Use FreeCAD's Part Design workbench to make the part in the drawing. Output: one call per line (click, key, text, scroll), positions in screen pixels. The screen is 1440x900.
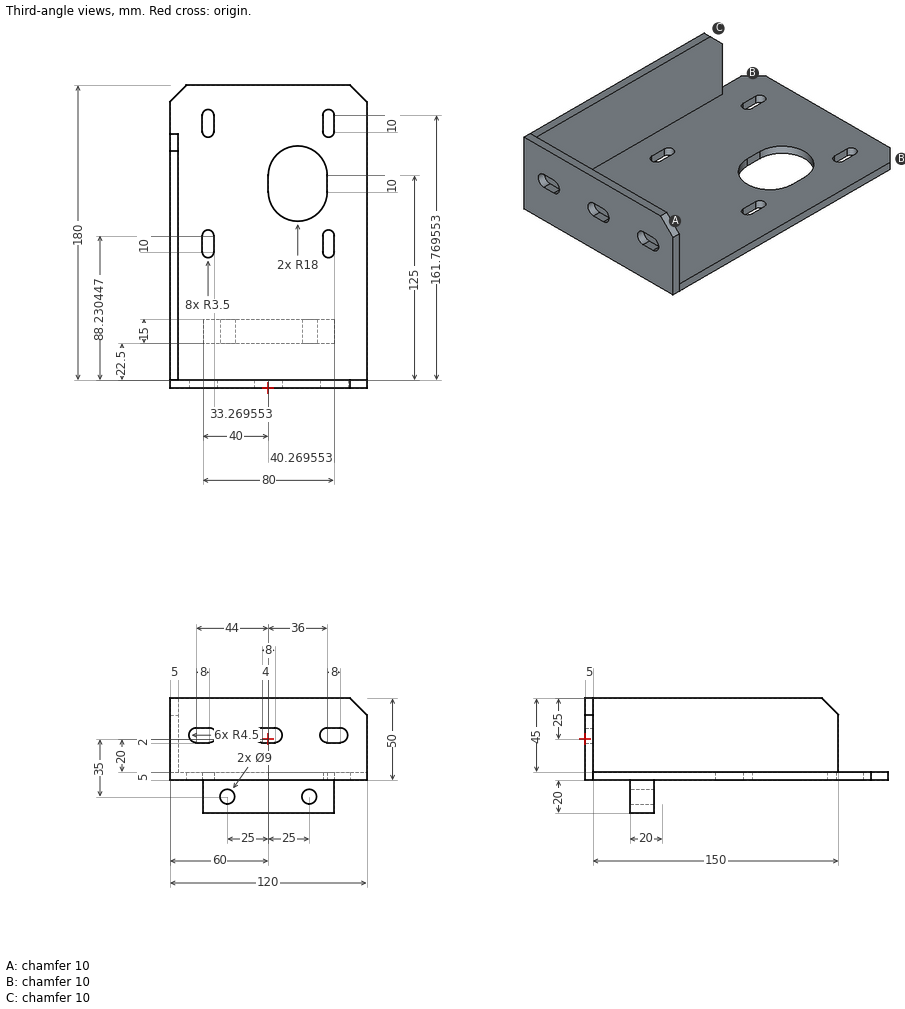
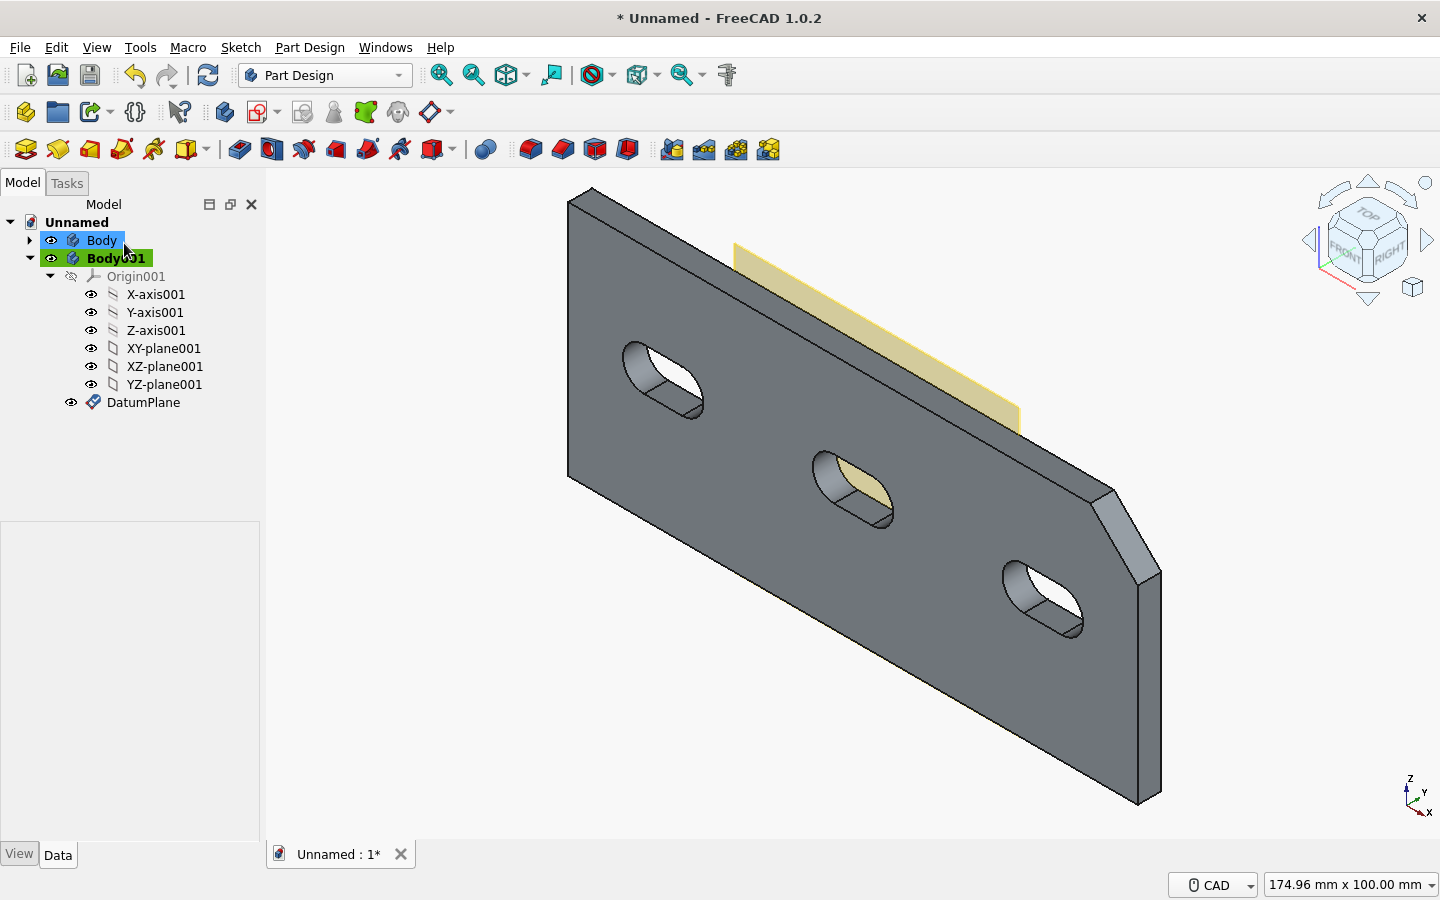
click(116, 402)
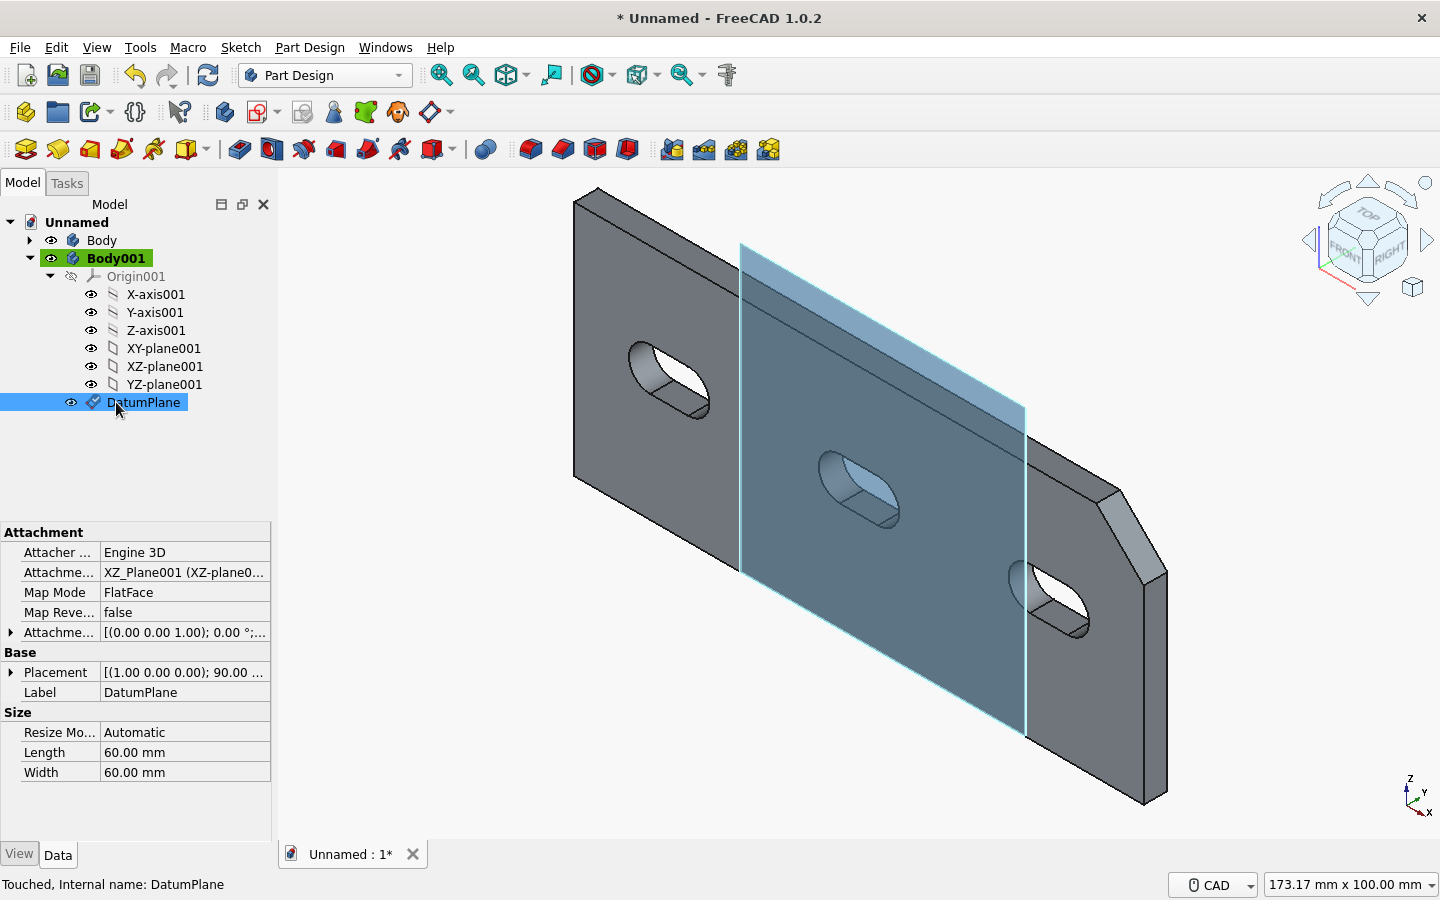
click(258, 112)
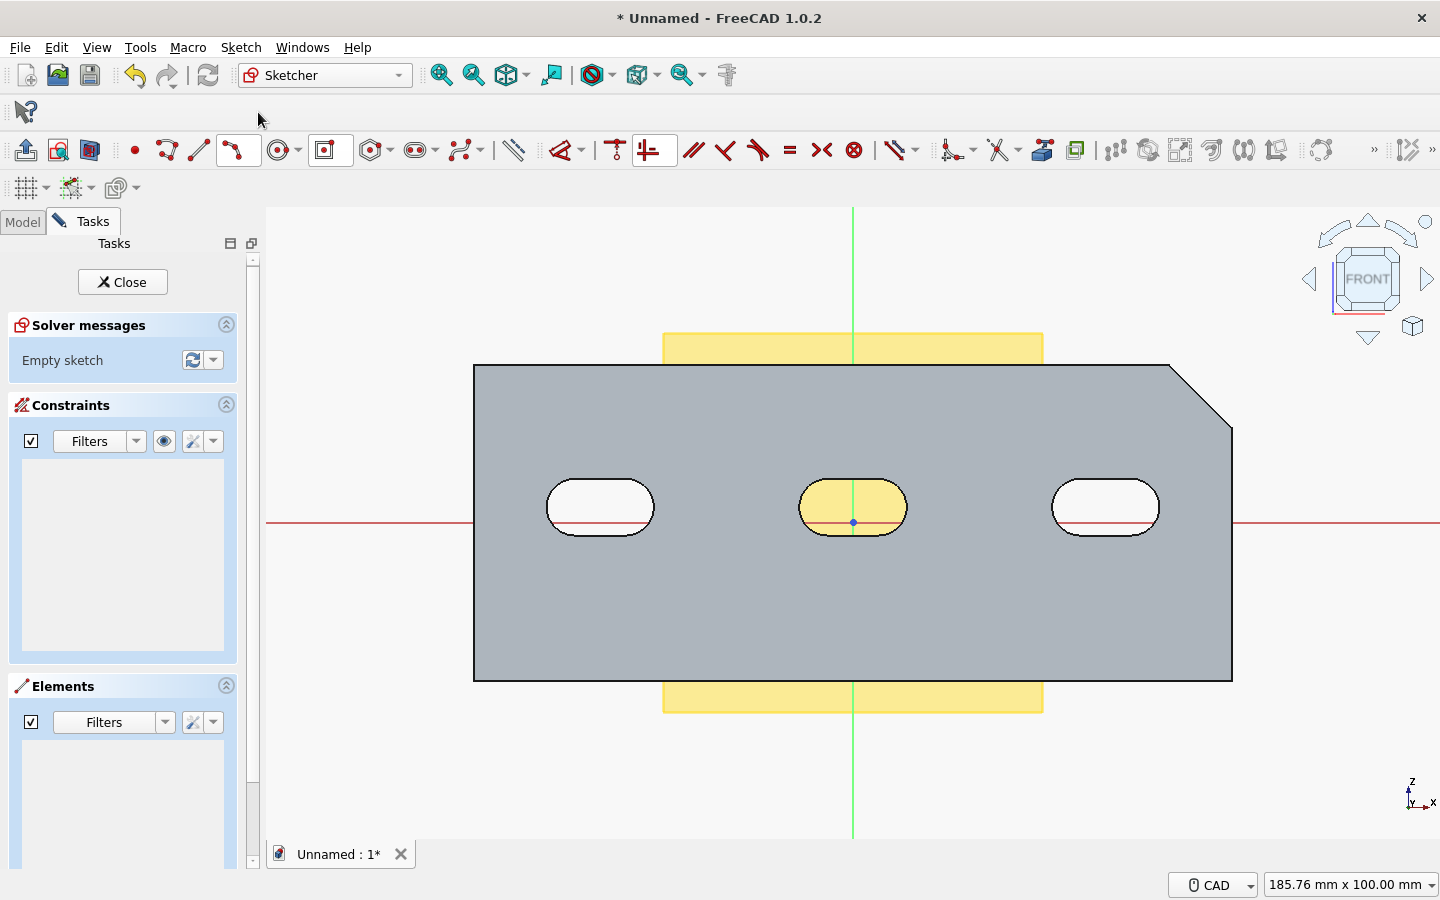
click(348, 150)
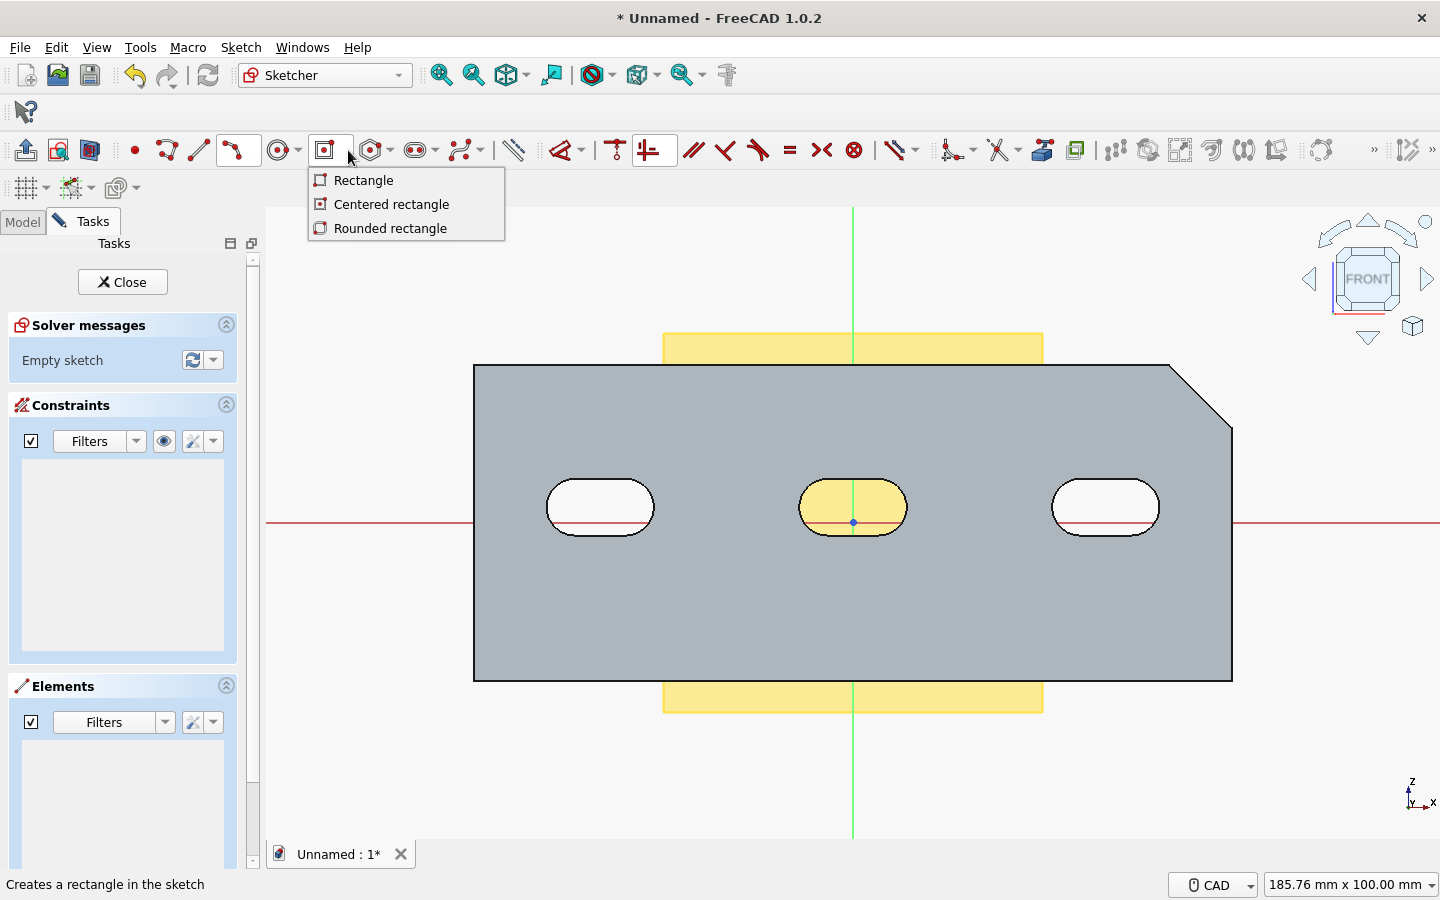
click(406, 180)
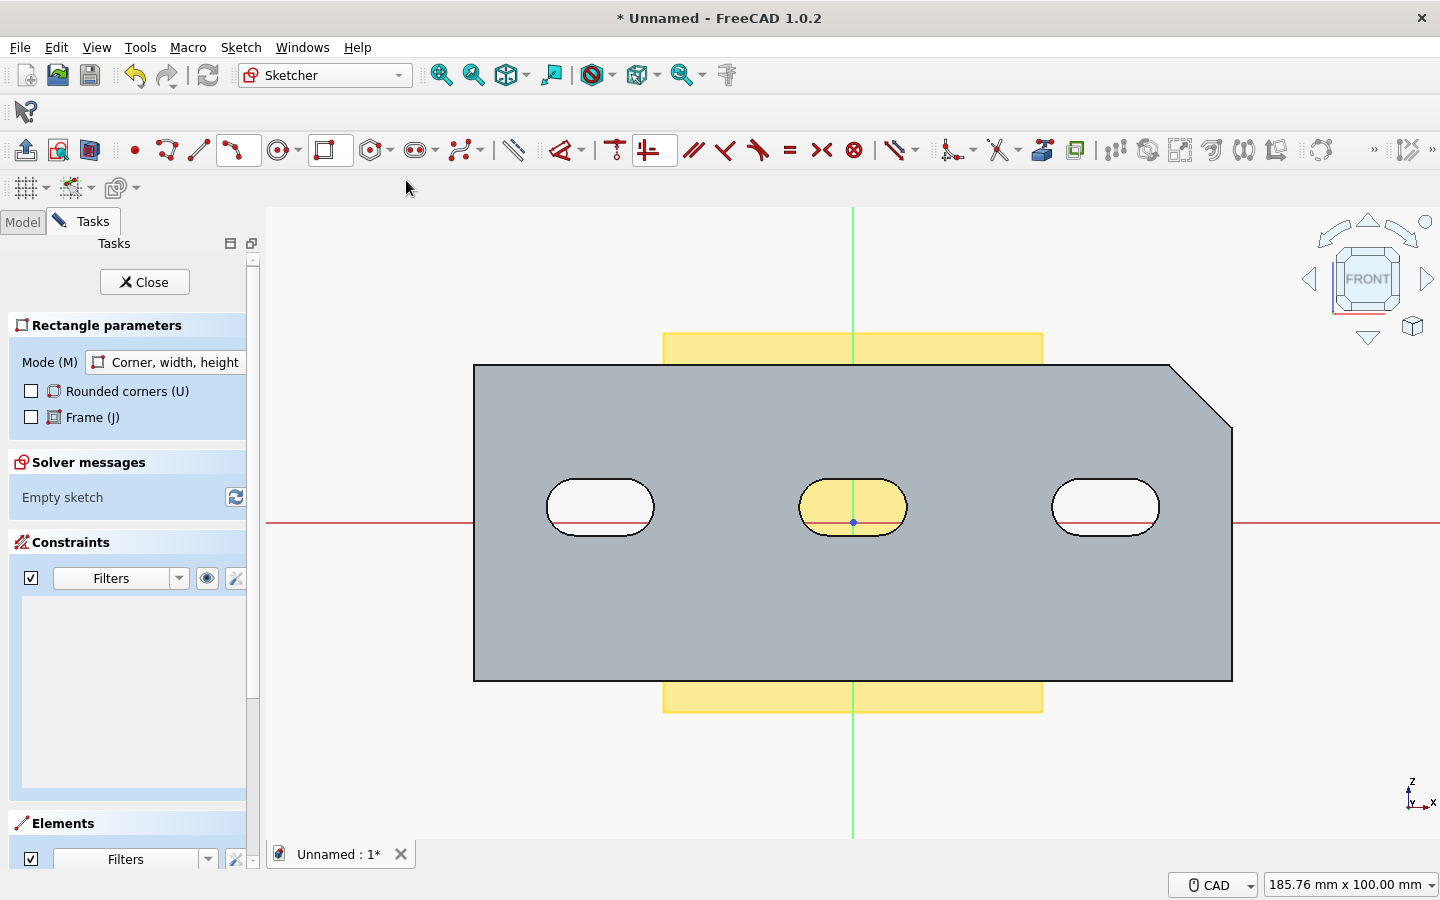
click(474, 649)
click(1232, 681)
key(Escape)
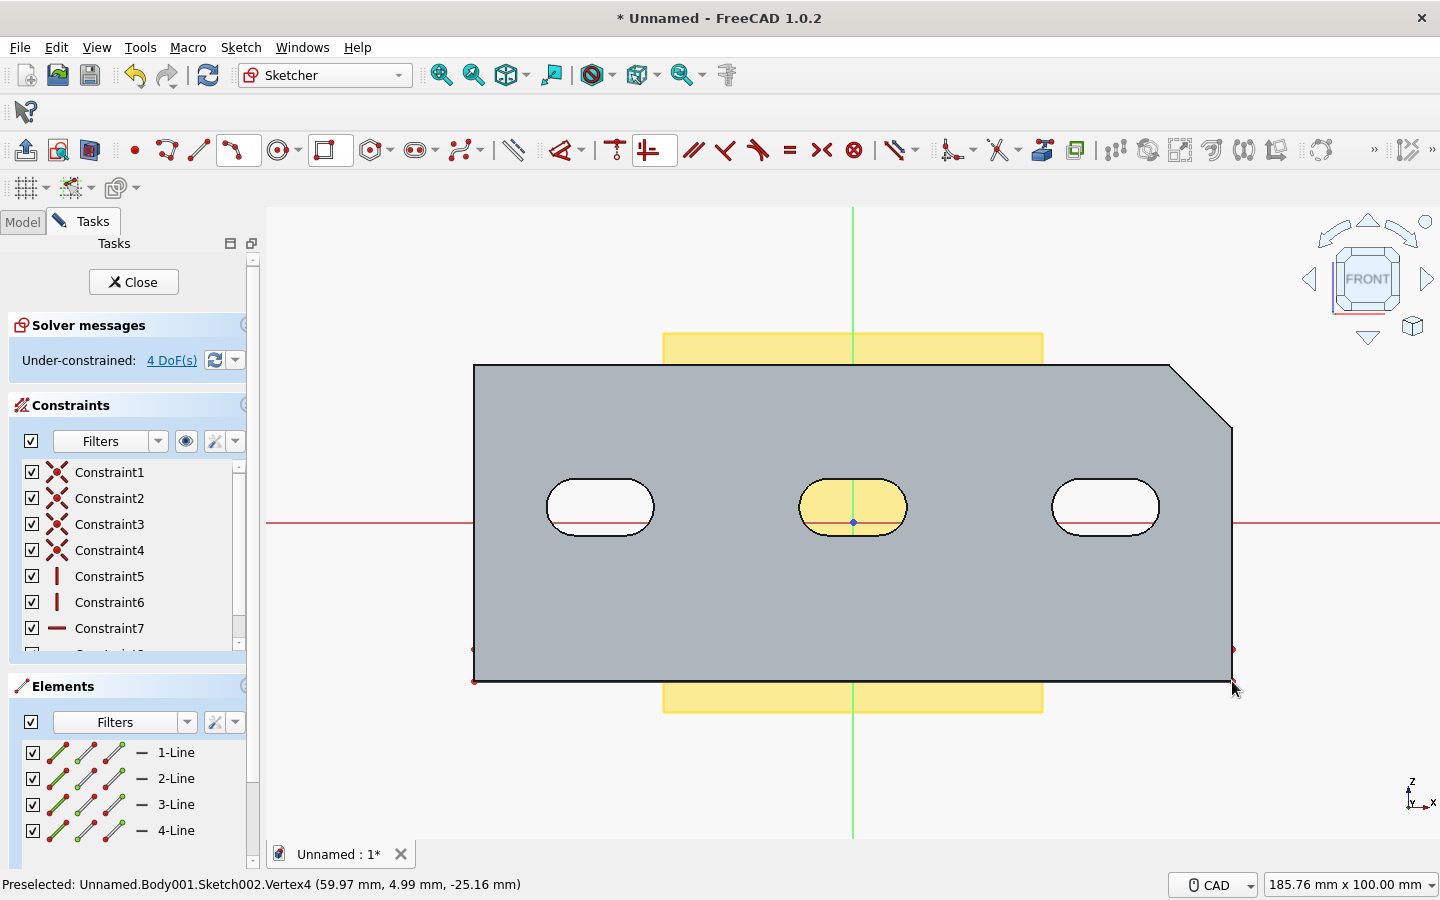
click(560, 150)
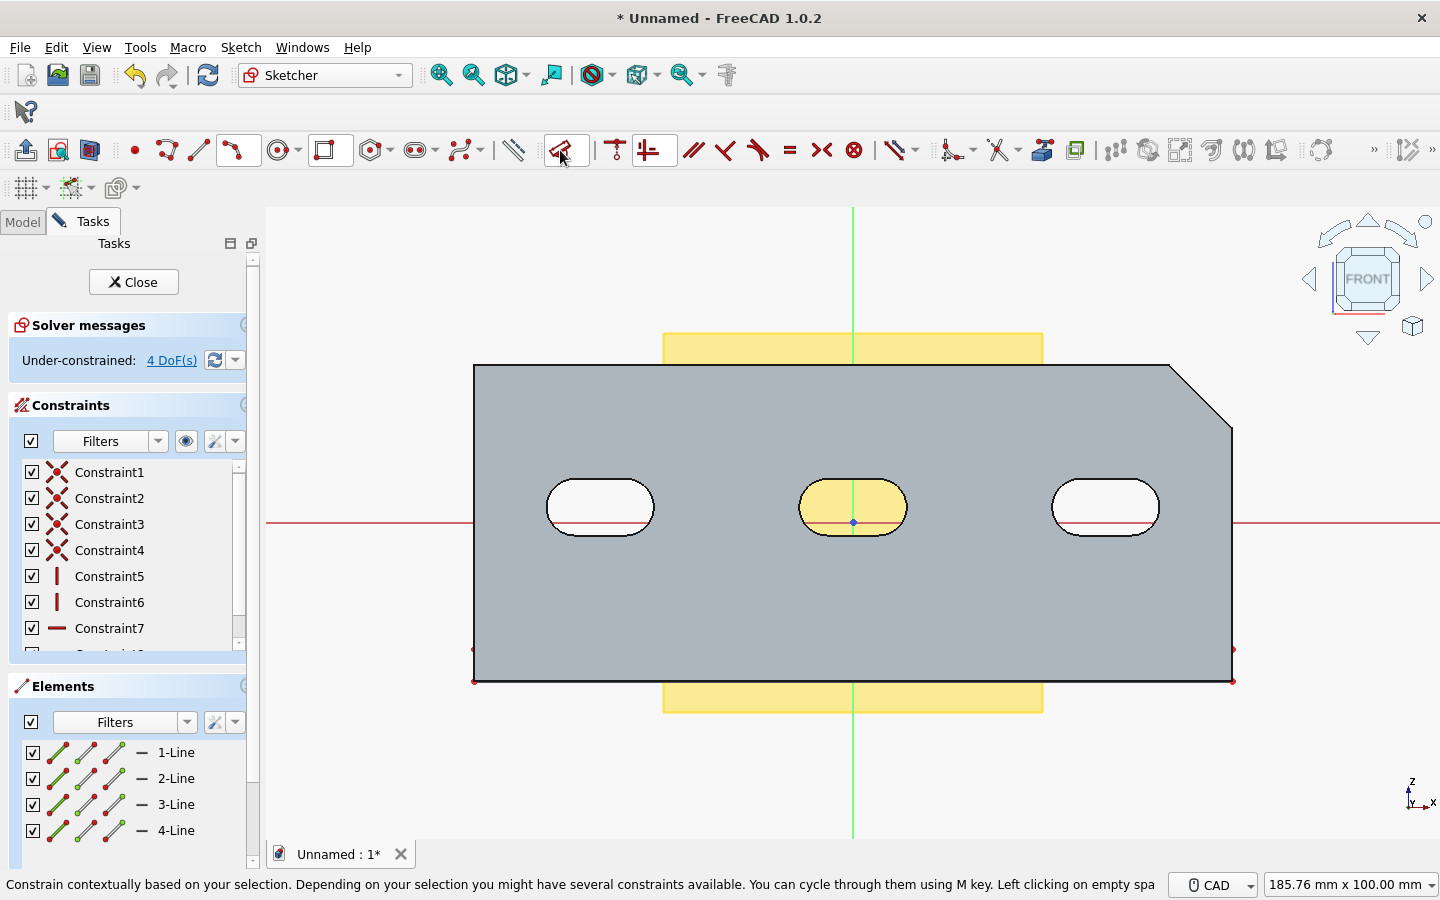
scroll(474, 660, up, 2)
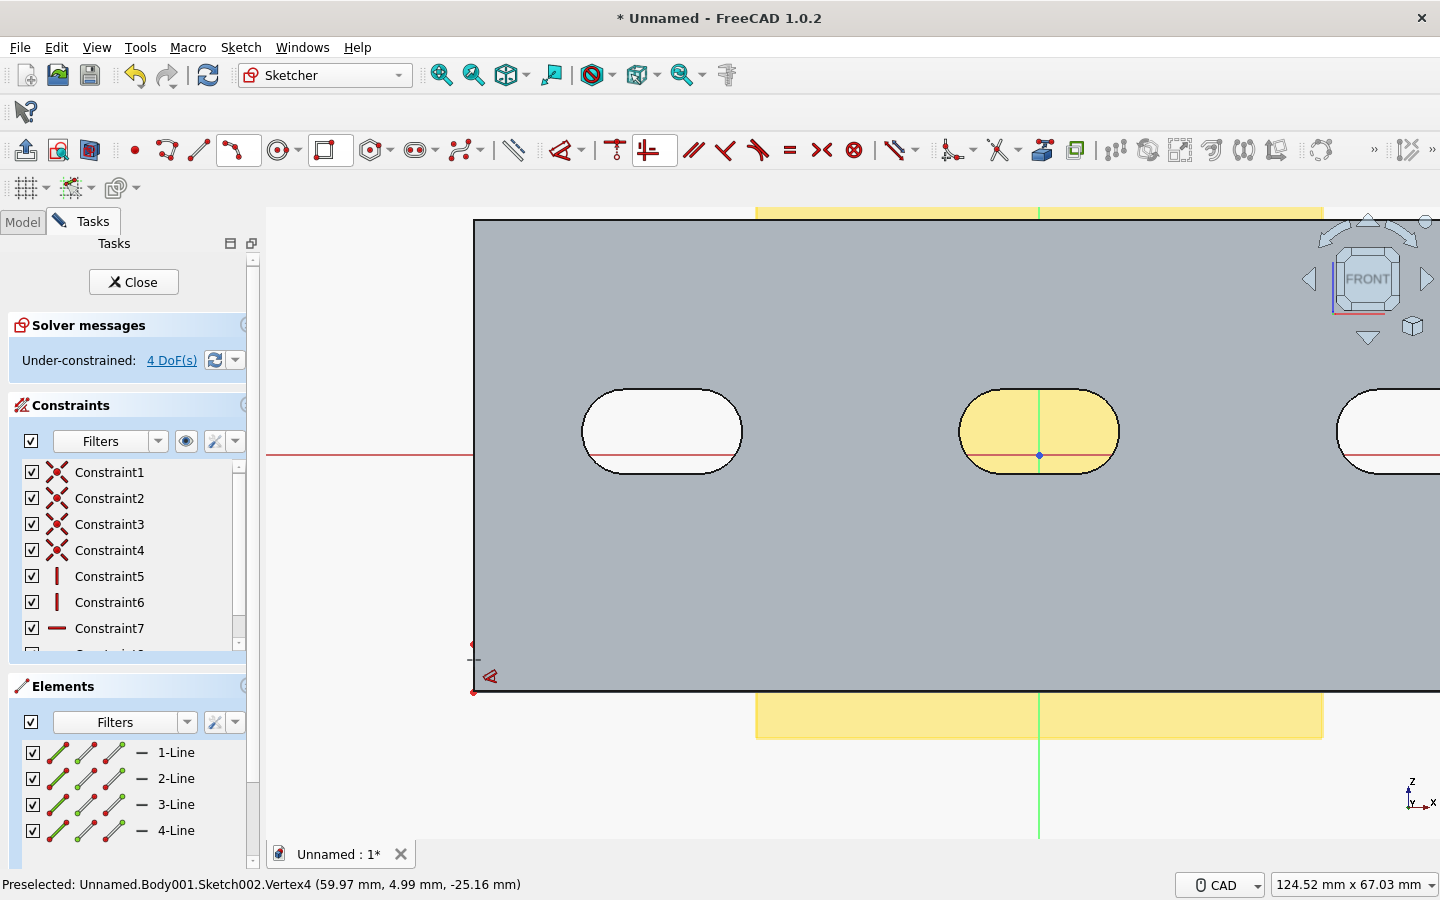
click(474, 659)
click(440, 669)